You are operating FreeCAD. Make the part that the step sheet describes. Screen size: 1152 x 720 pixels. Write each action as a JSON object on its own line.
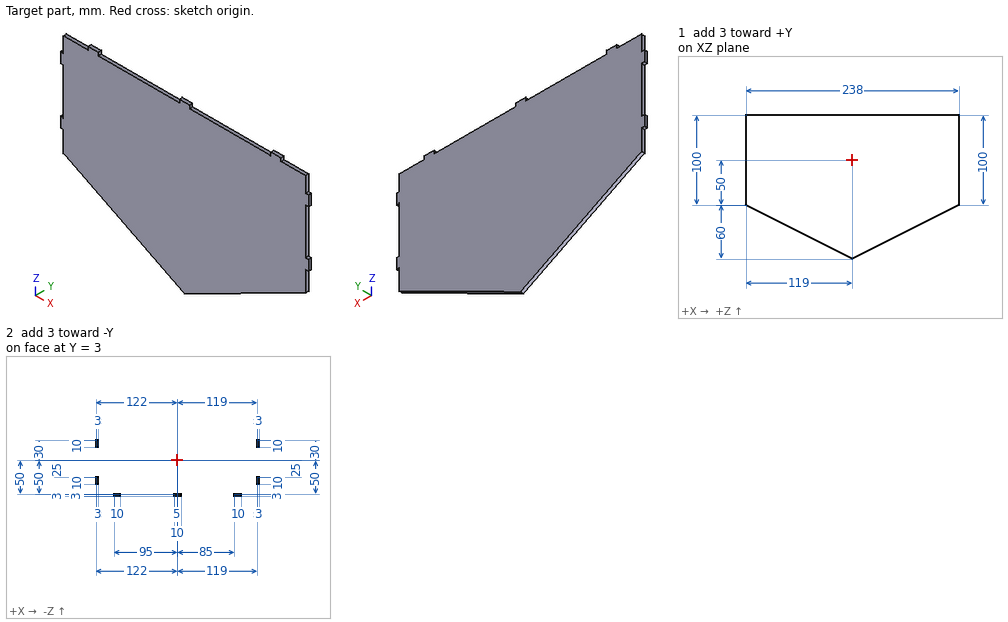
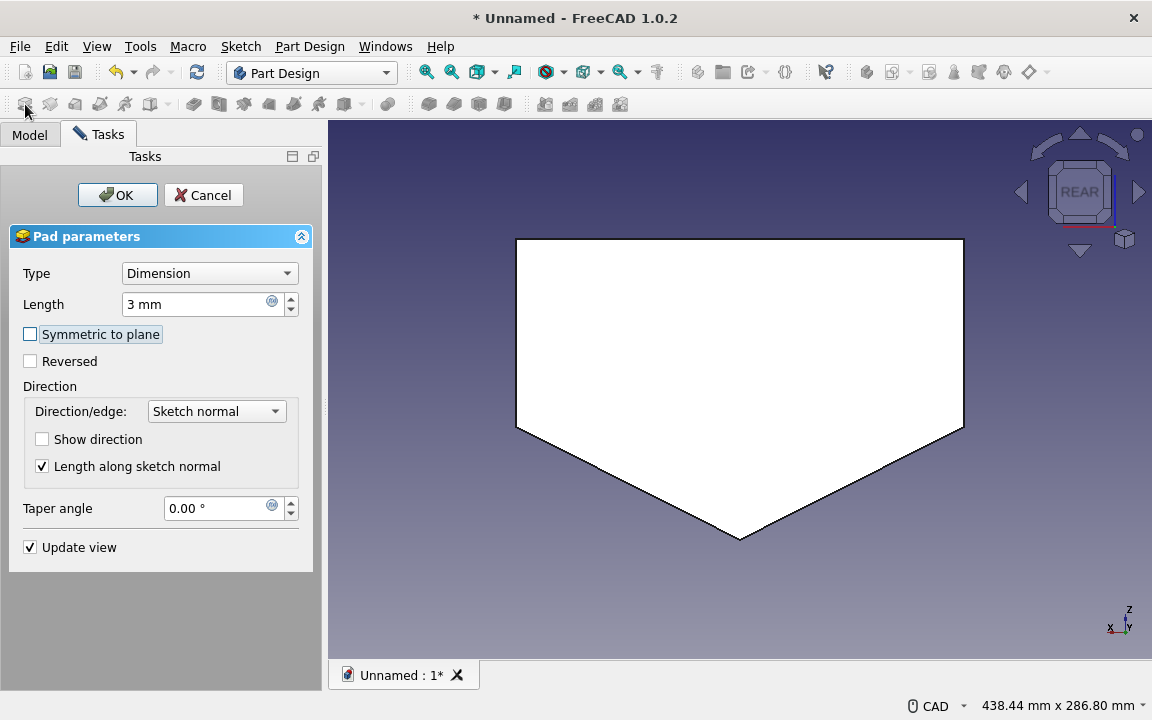
{"action": "left_click", "coordinate": [31, 361]}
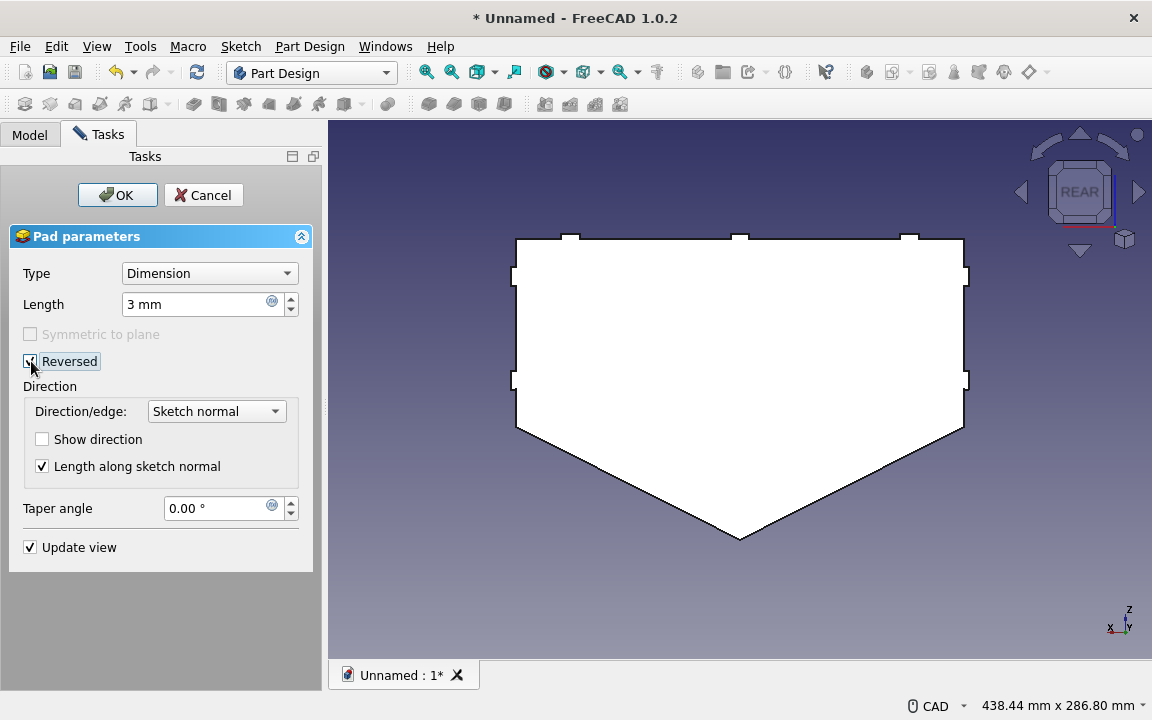
{"action": "left_click", "coordinate": [118, 195]}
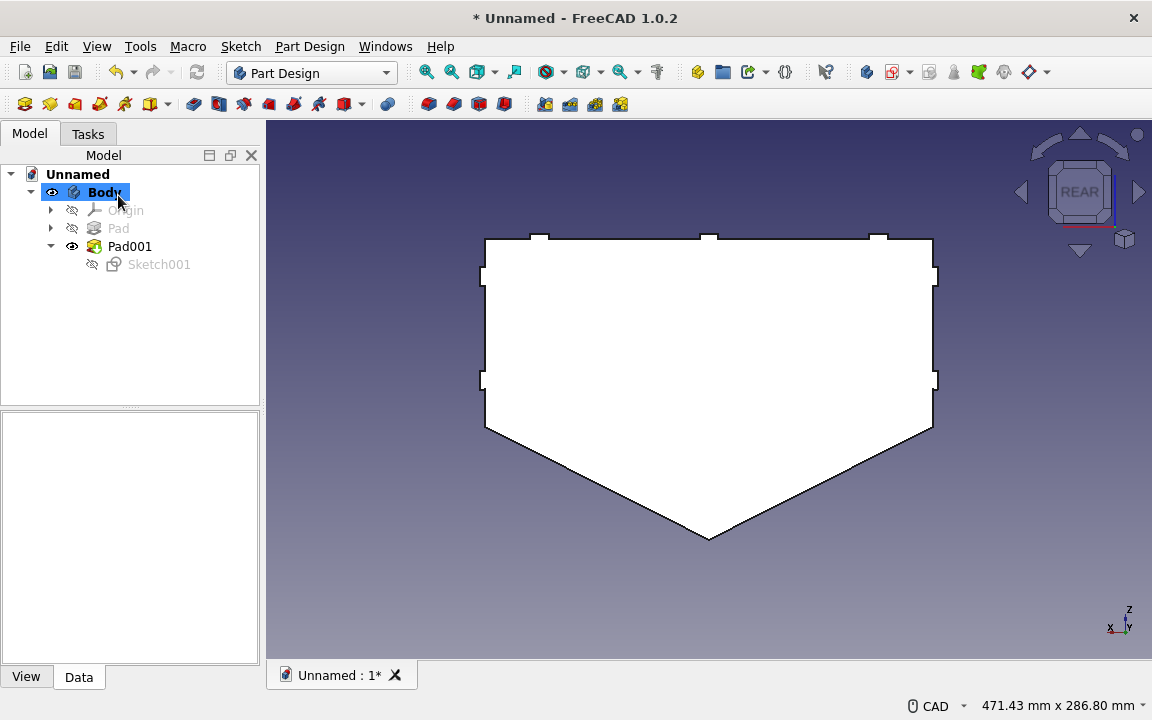
{"action": "key", "text": "0"}